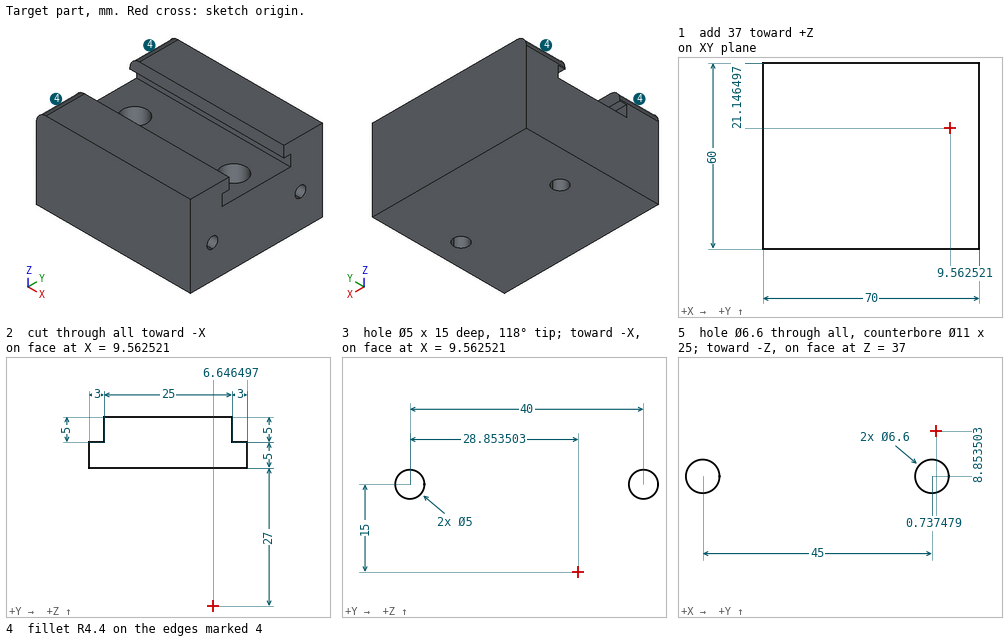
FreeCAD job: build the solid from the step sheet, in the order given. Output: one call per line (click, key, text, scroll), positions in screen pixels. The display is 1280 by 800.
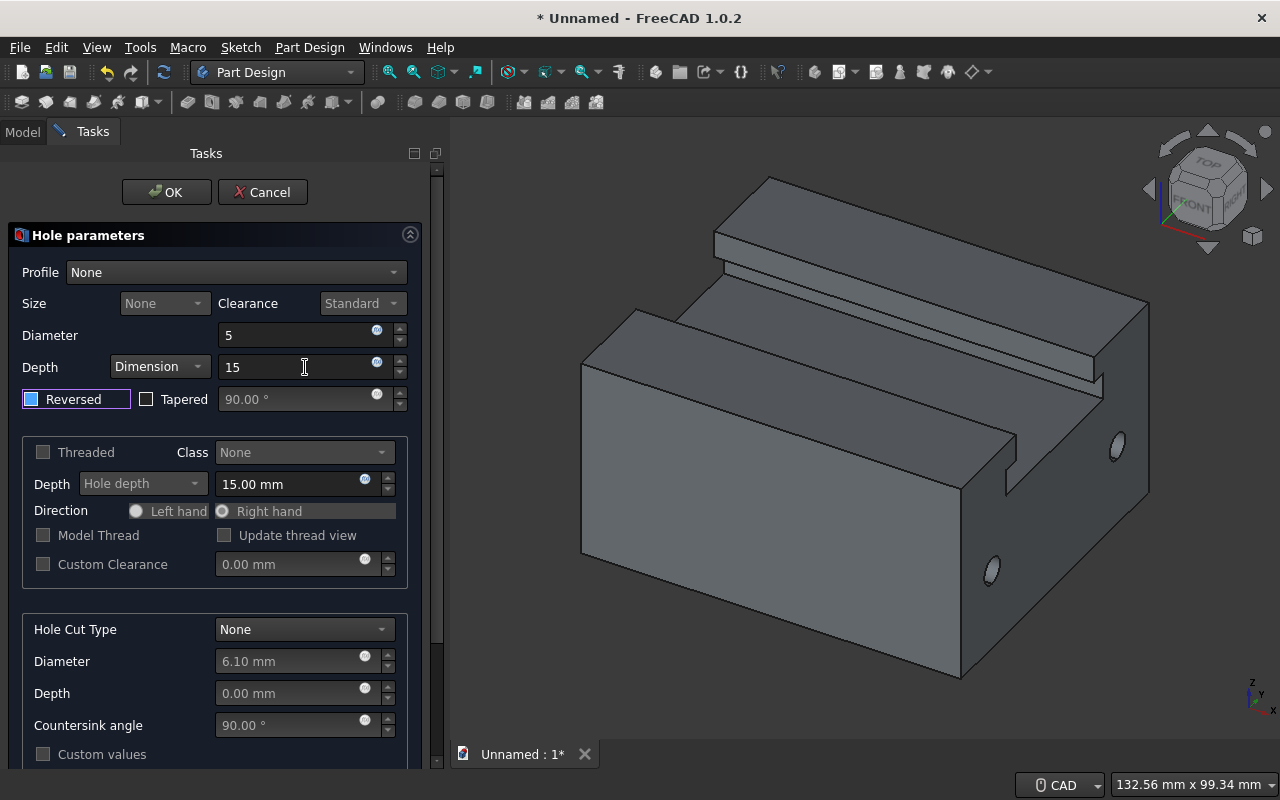
click(167, 192)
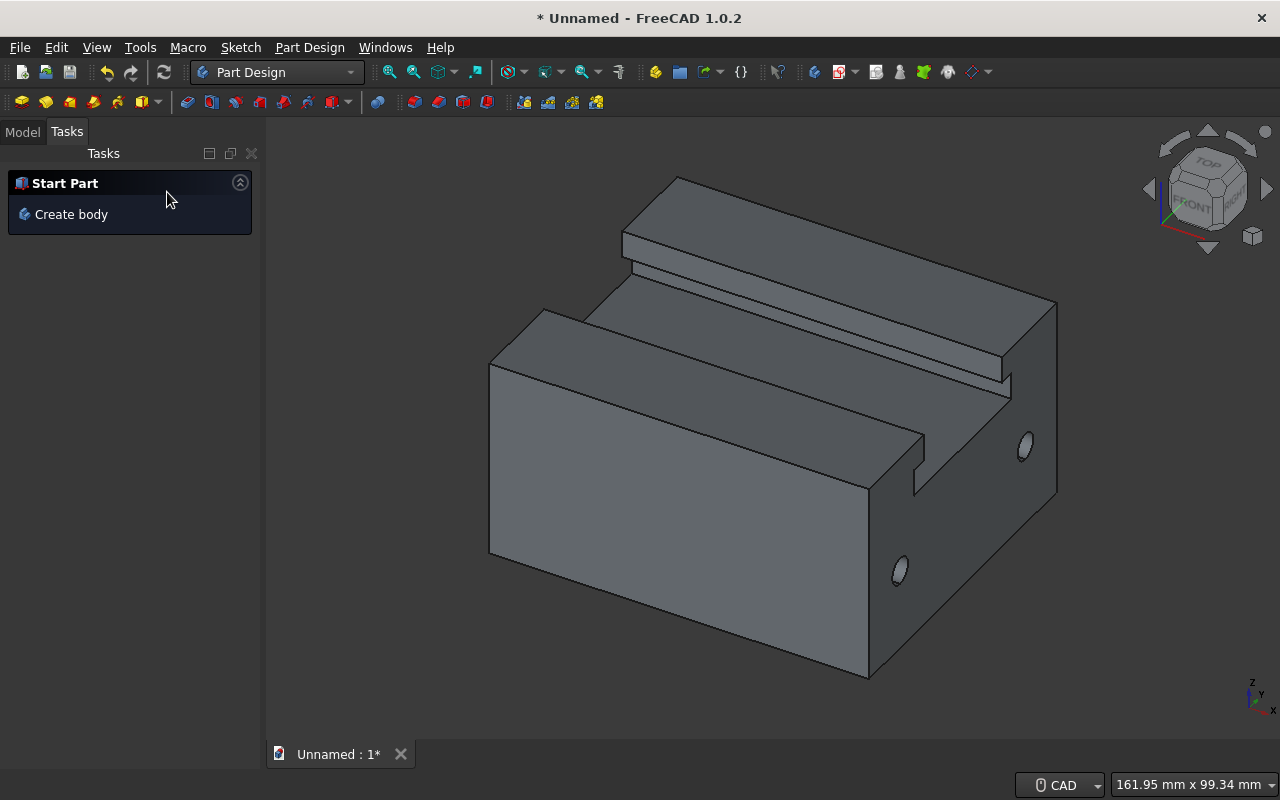
key(0)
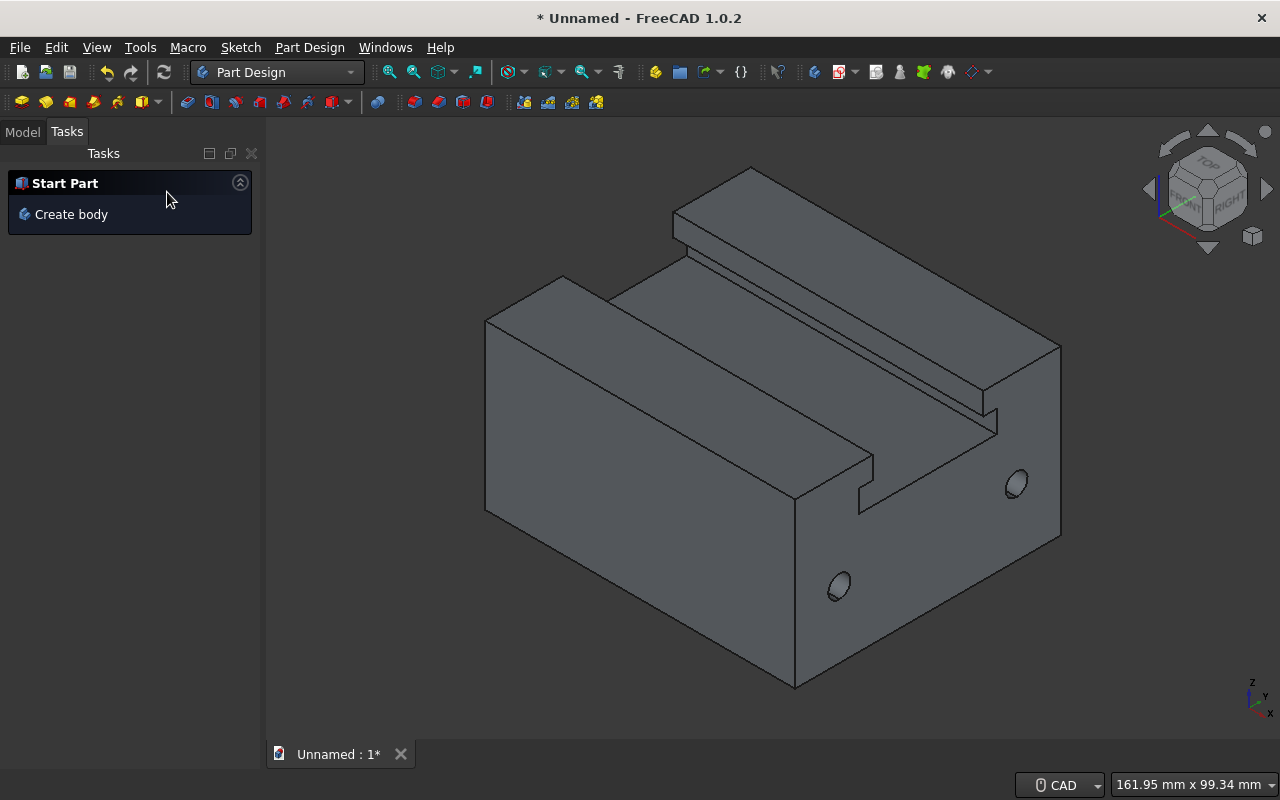
key(2)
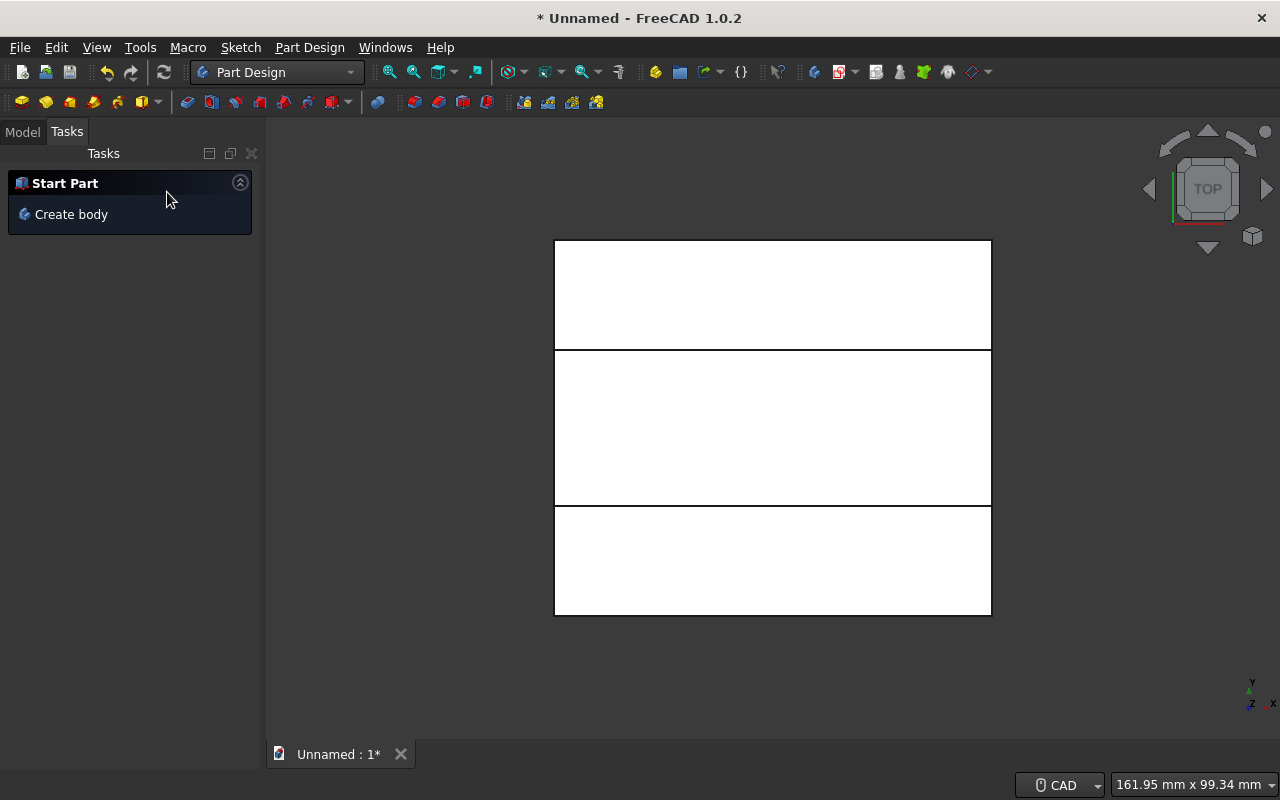
click(554, 560)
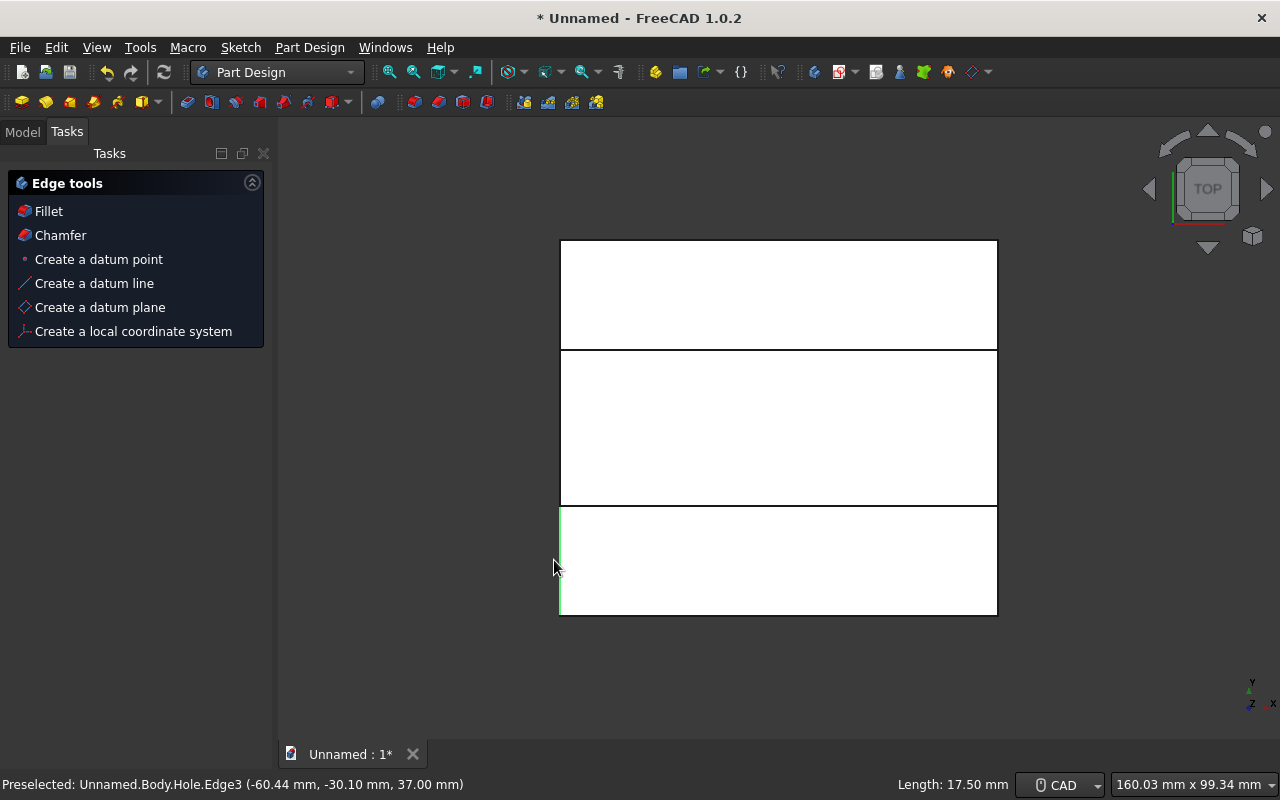
click(560, 294, ctrl)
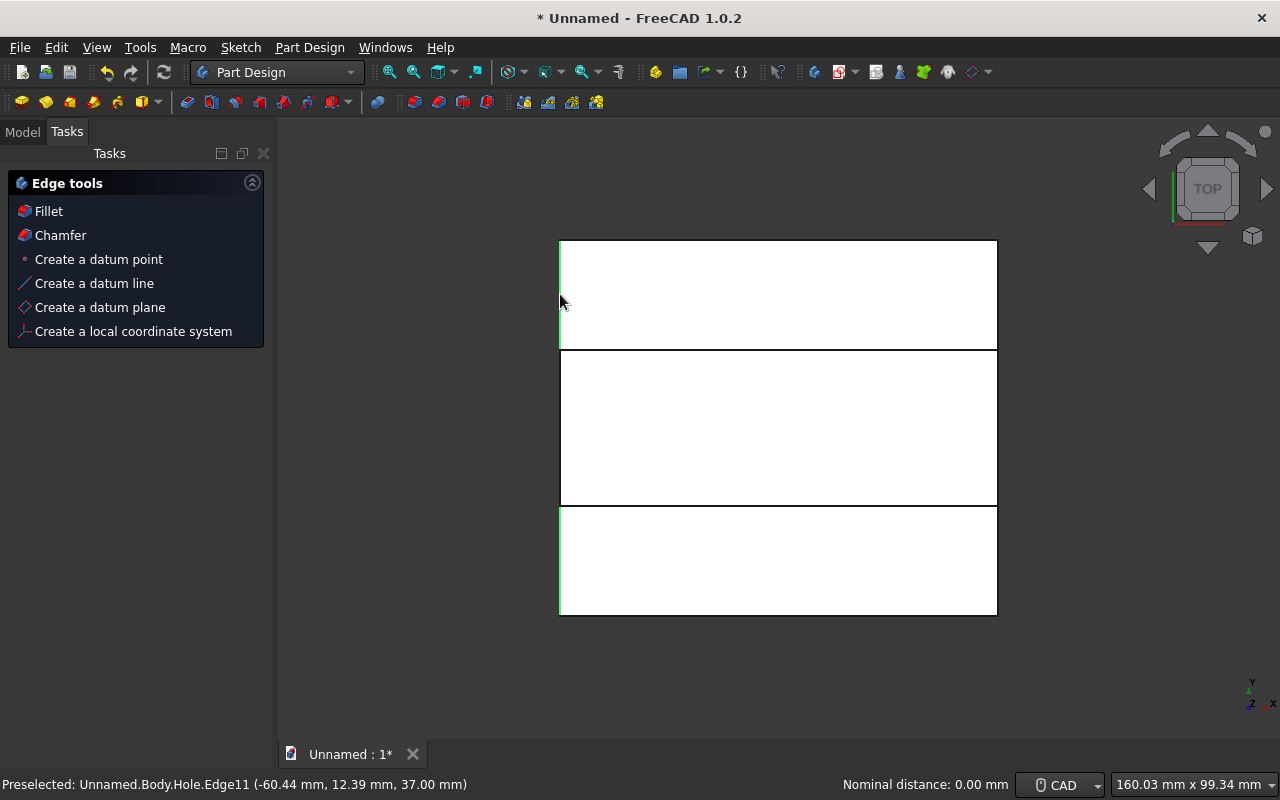
click(416, 102)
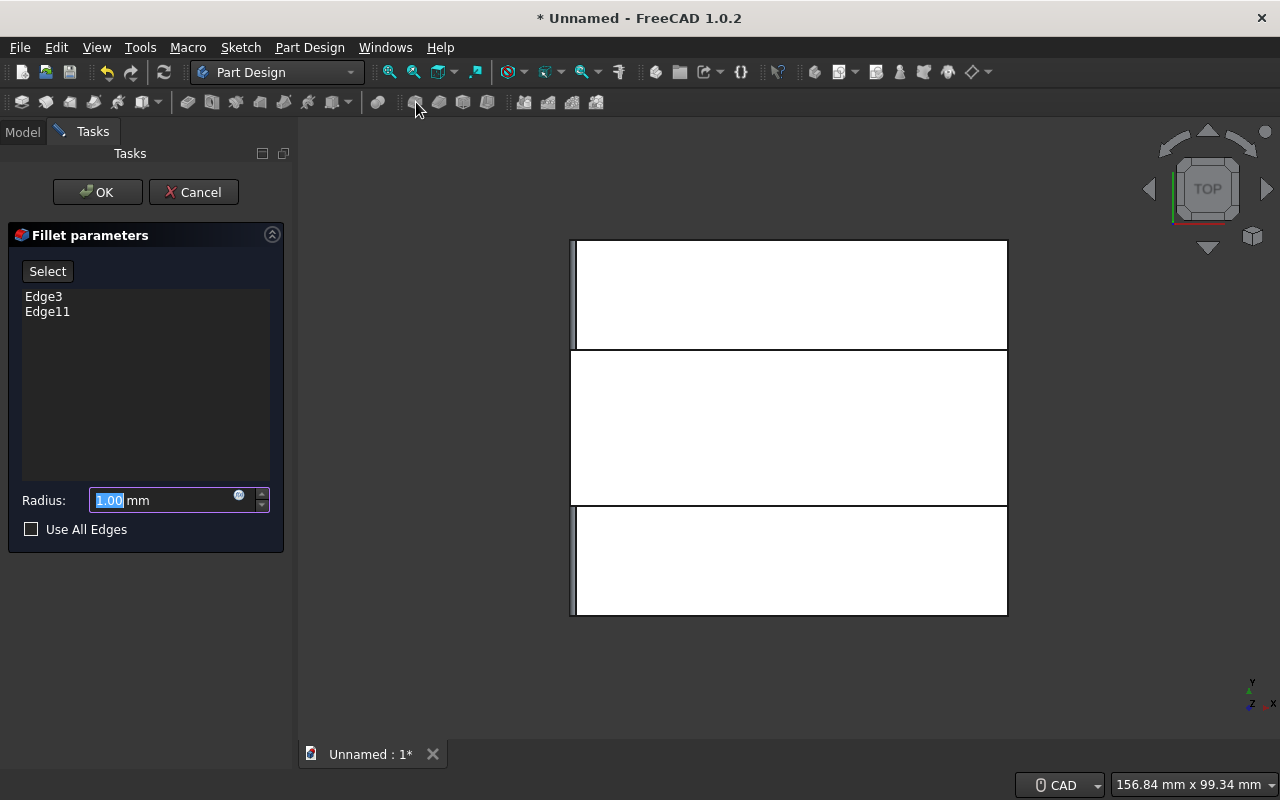
text(4.4)
key(Tab)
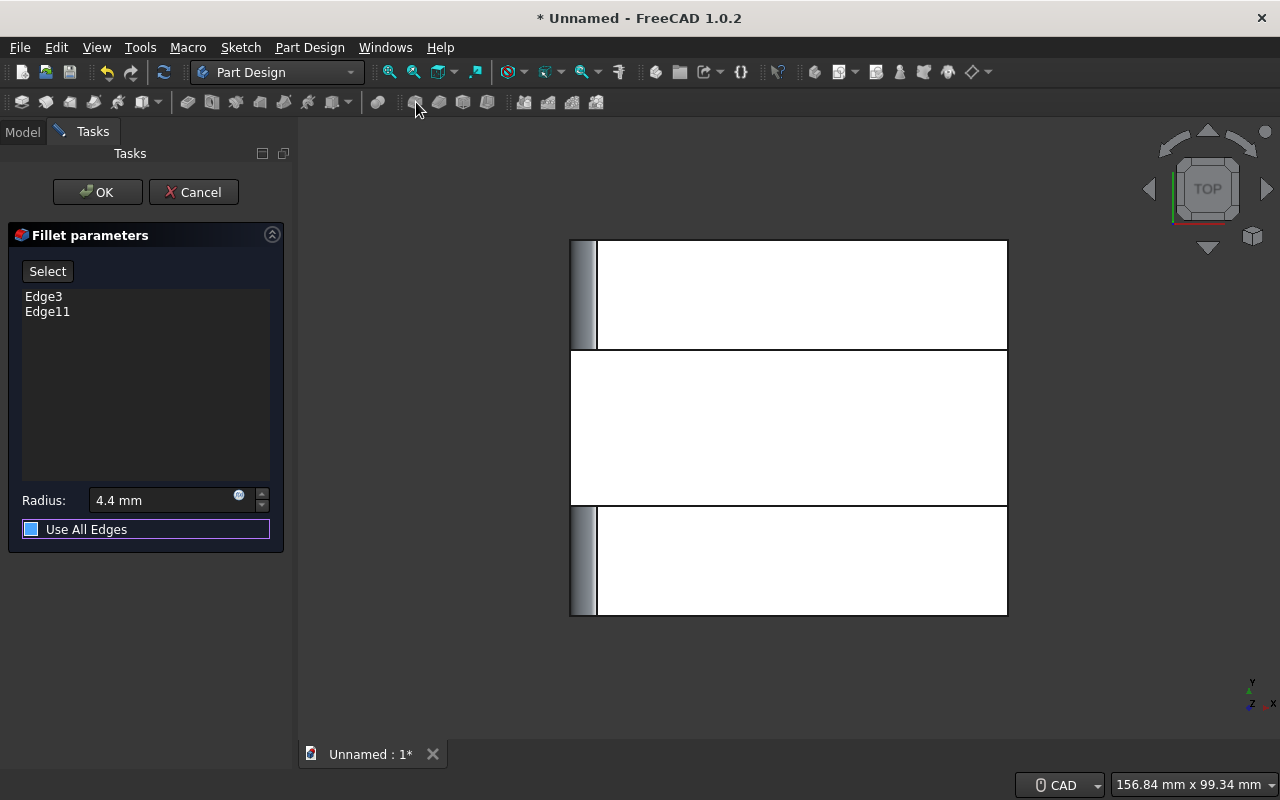
click(98, 192)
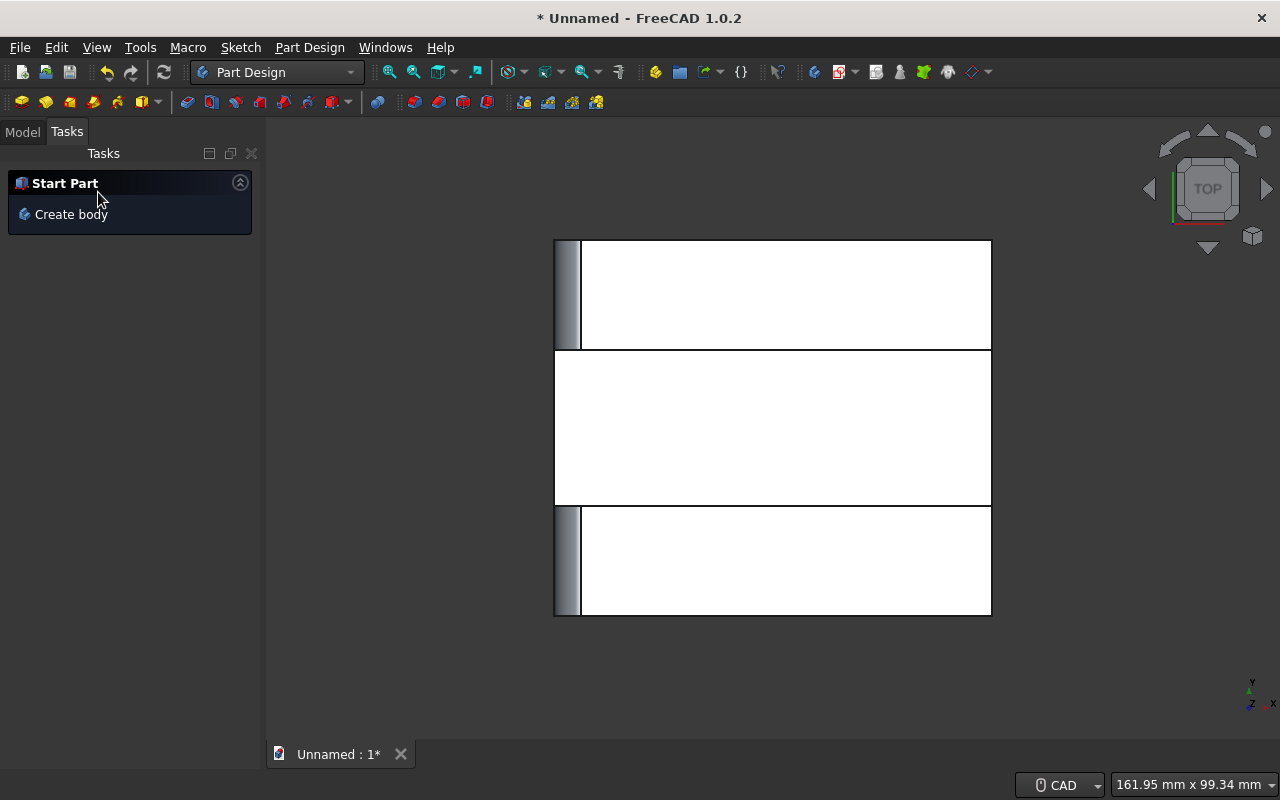
click(904, 294)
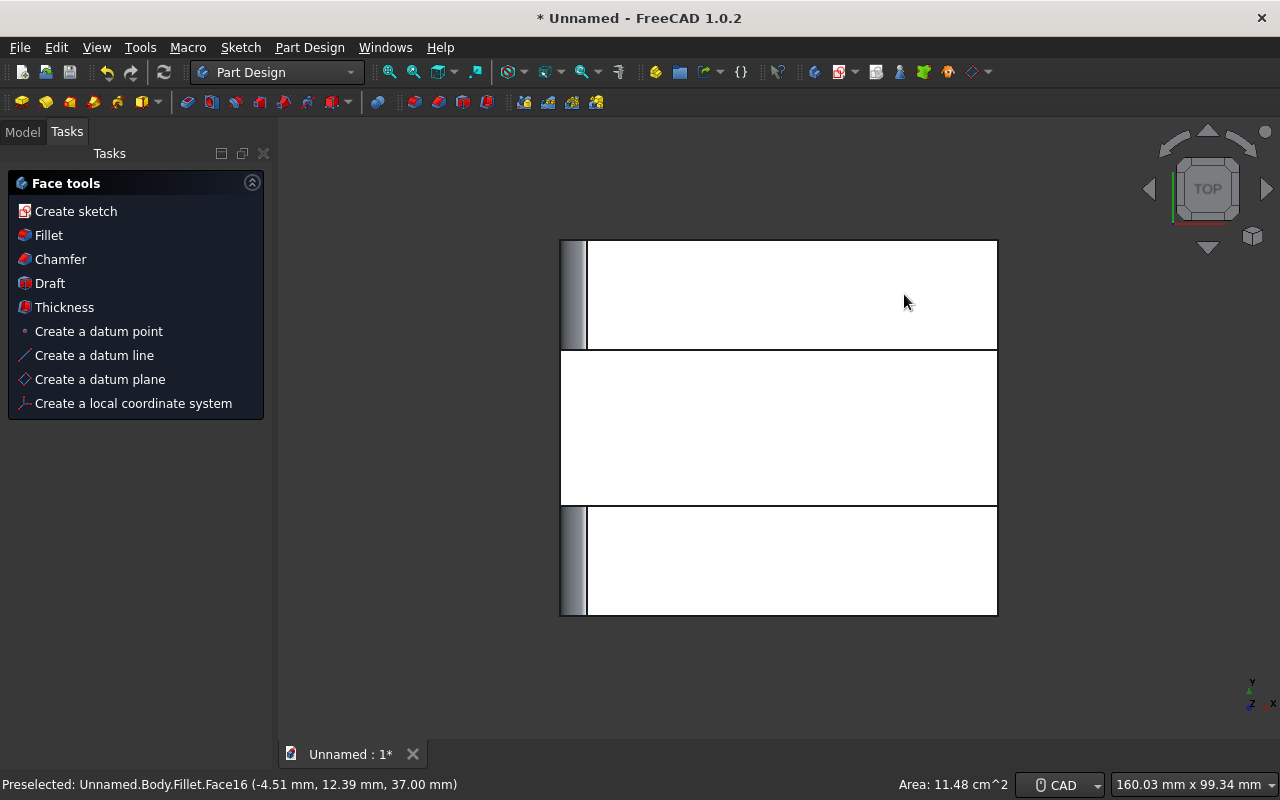
click(840, 72)